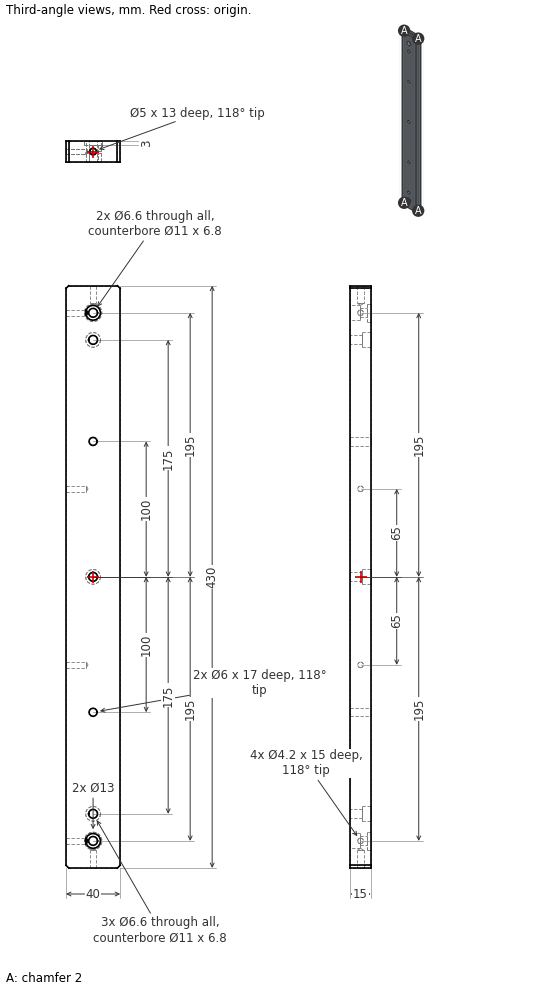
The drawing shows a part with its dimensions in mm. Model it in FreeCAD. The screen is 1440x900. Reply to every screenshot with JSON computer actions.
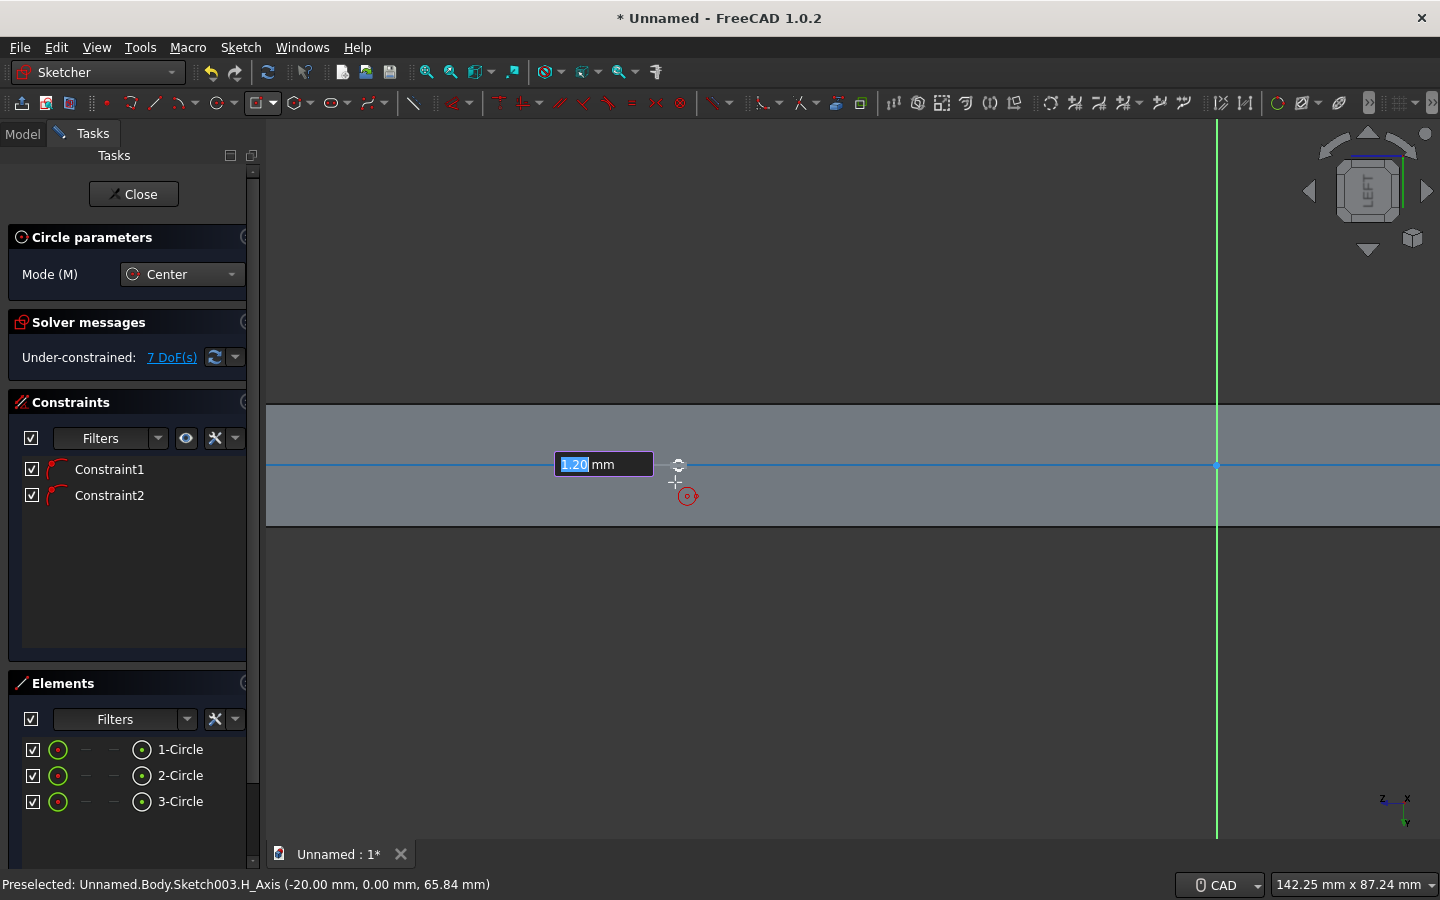
{"action": "left_click", "coordinate": [675, 482]}
{"action": "key", "text": "Escape"}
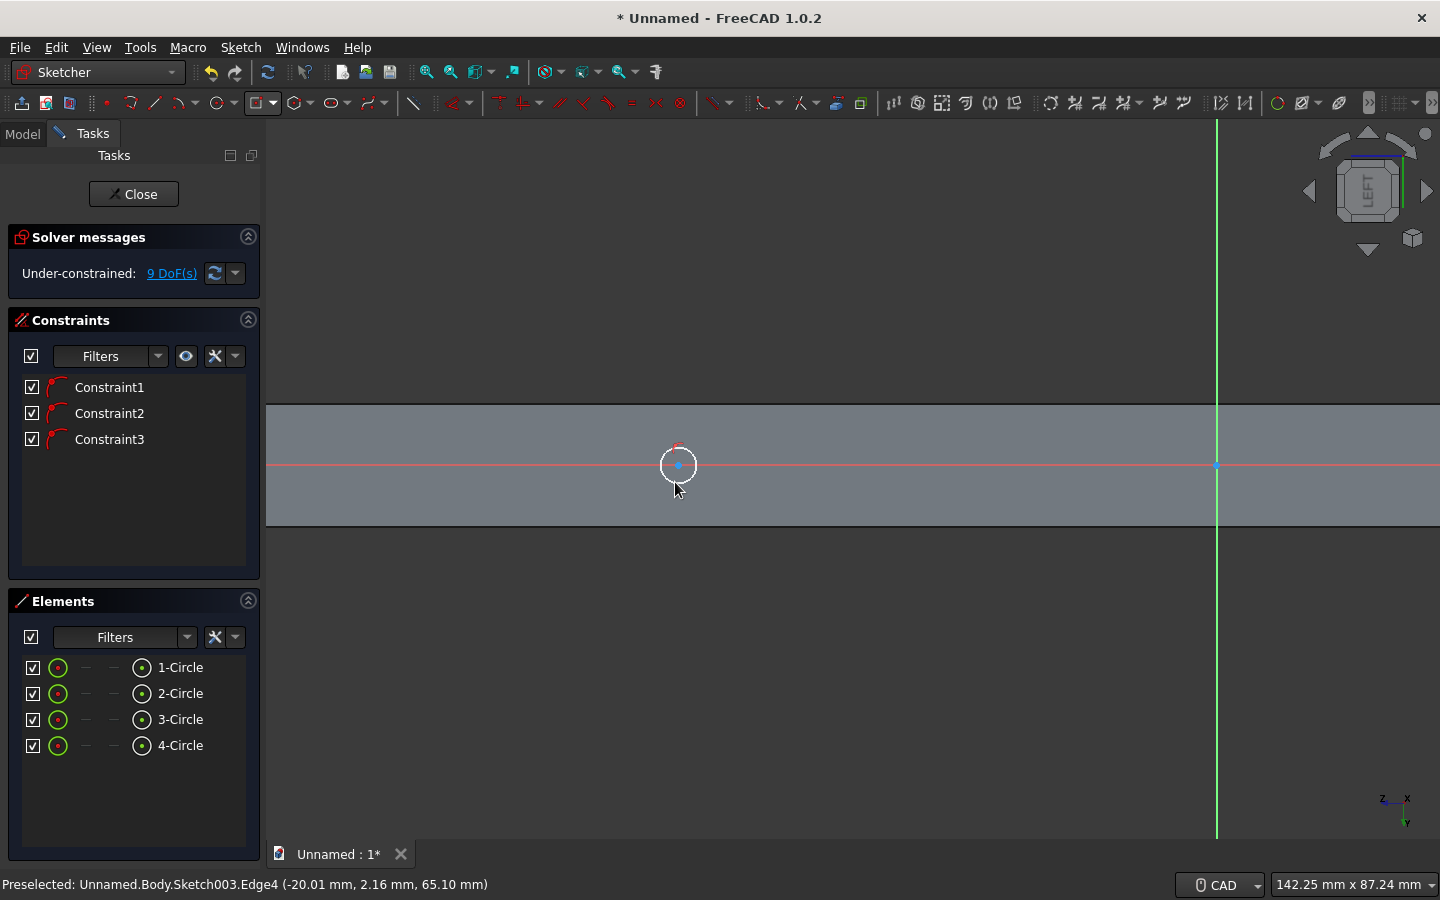
{"action": "scroll", "coordinate": [675, 482], "scroll_direction": "down", "scroll_amount": 8}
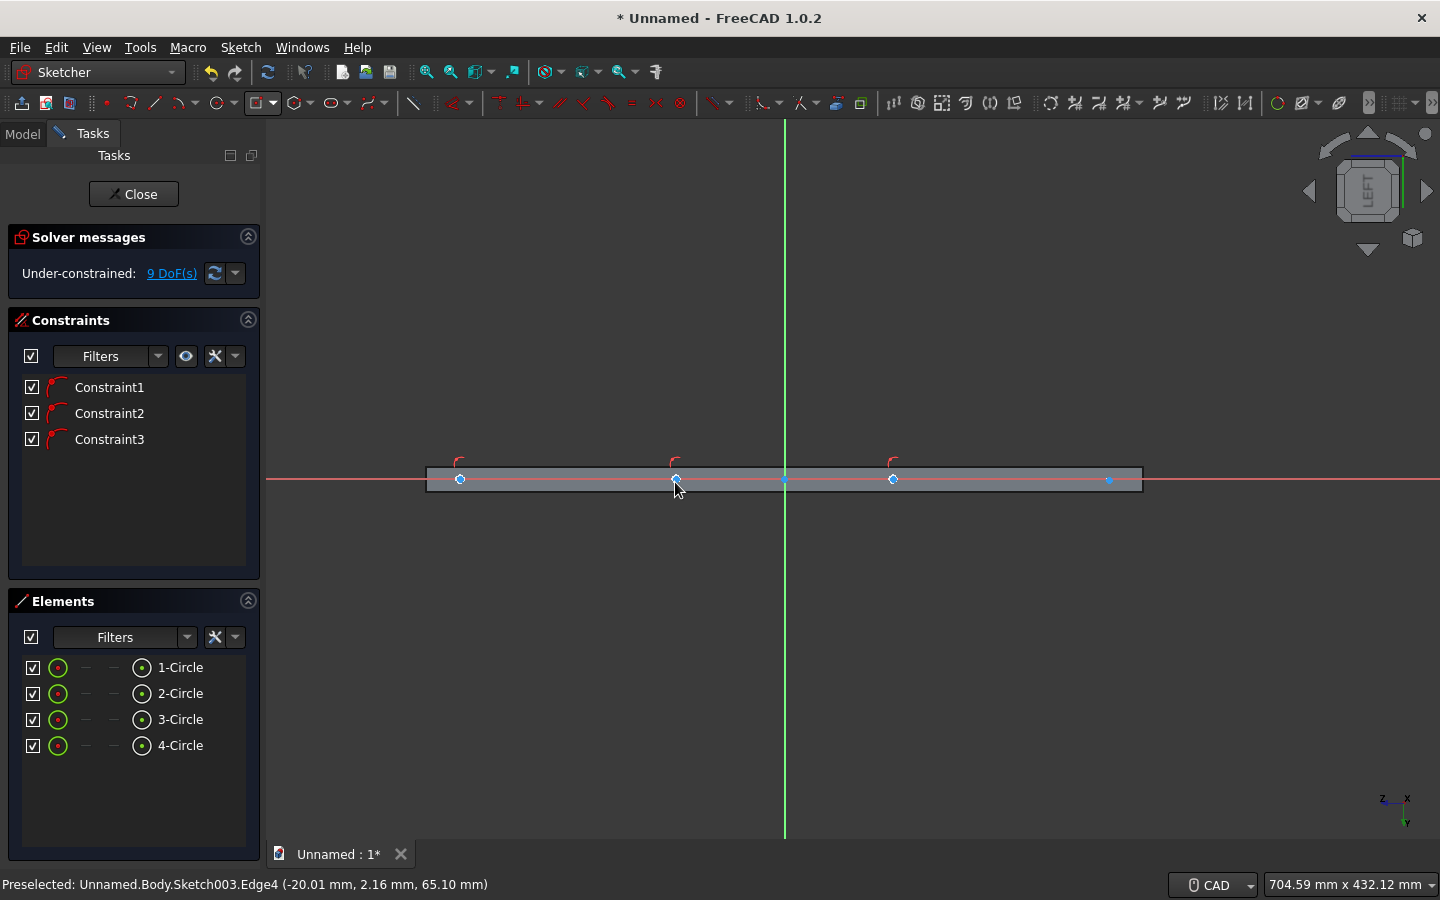
{"action": "scroll", "coordinate": [1111, 478], "scroll_direction": "up", "scroll_amount": 9}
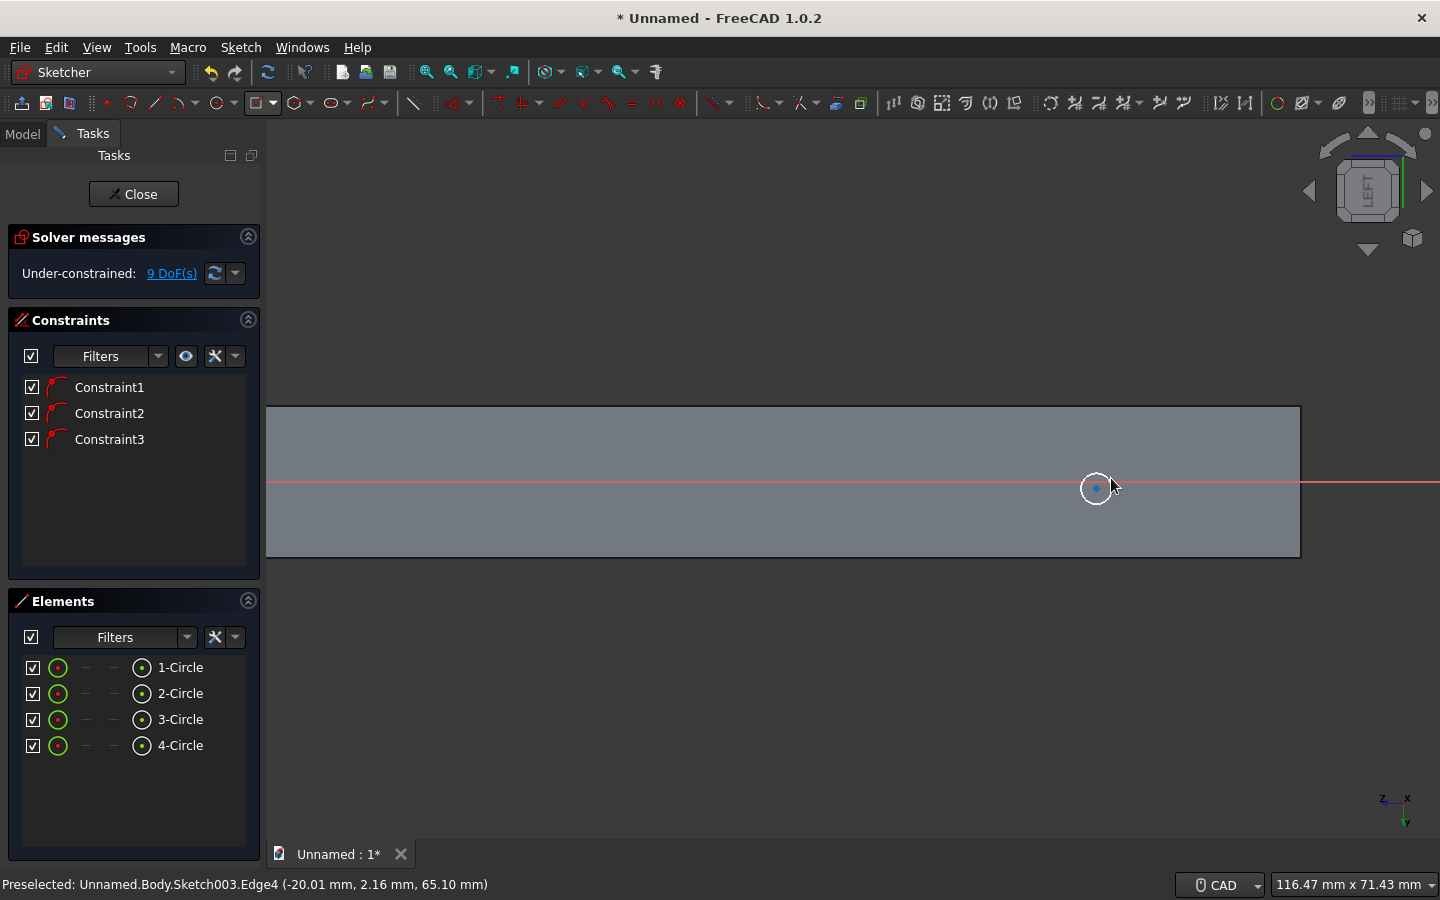
{"action": "left_click", "coordinate": [1107, 478]}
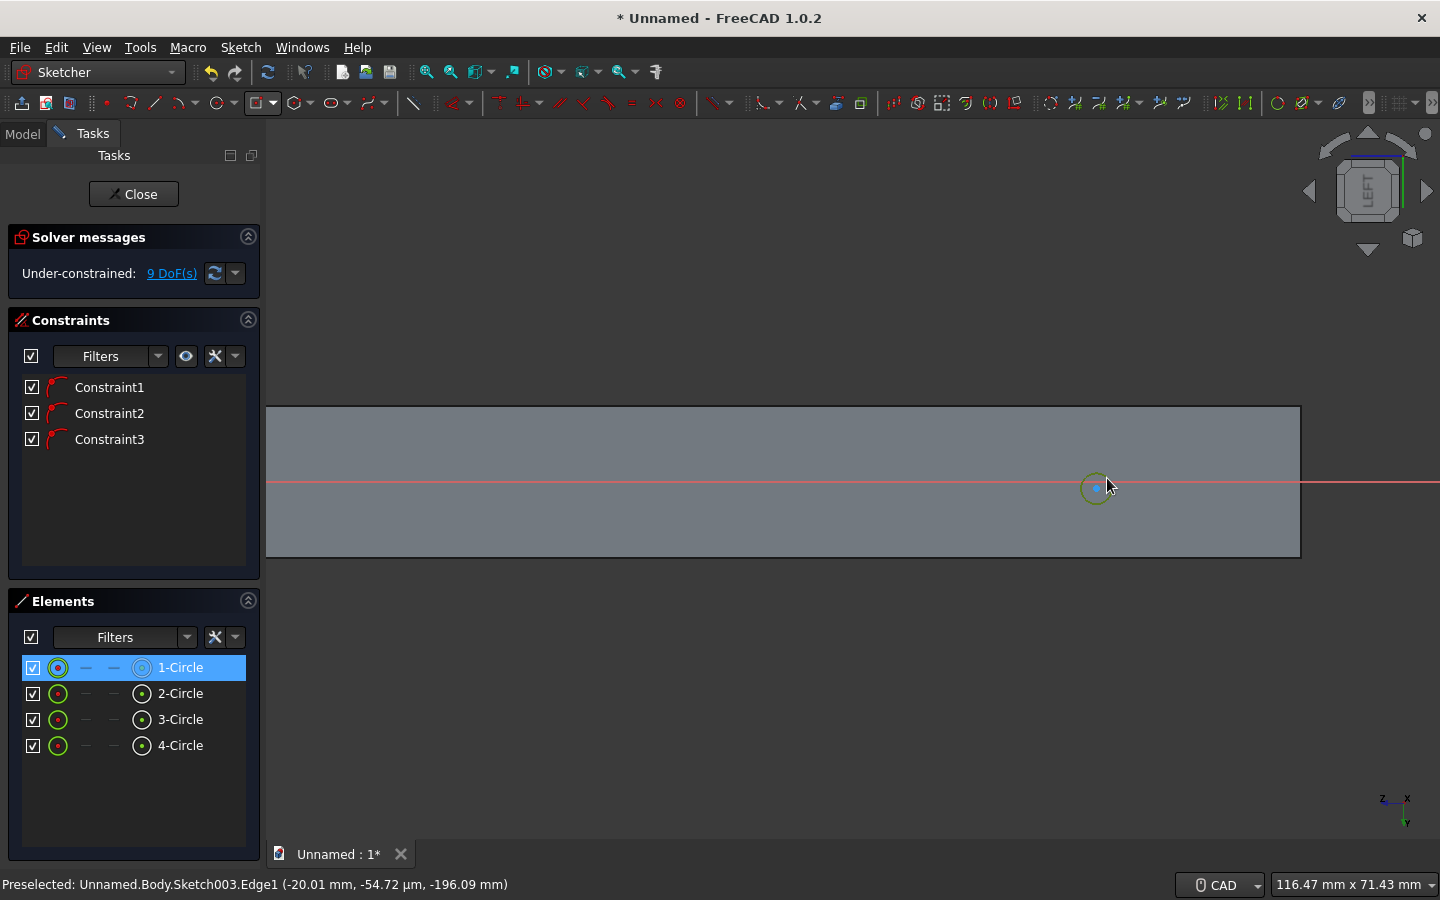
{"action": "scroll", "coordinate": [1111, 478], "scroll_direction": "down", "scroll_amount": 9}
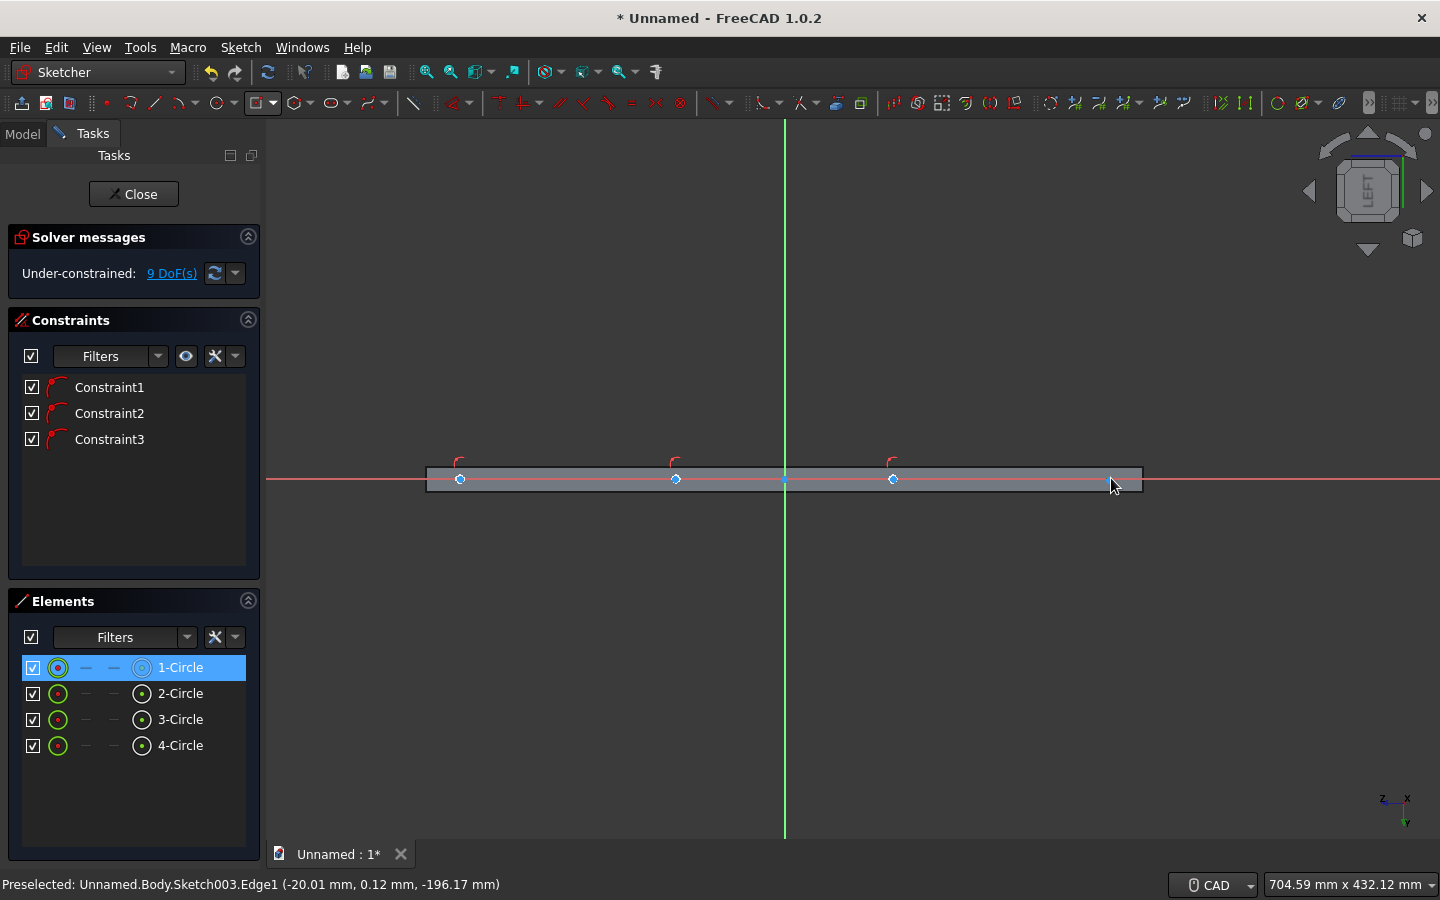
{"action": "scroll", "coordinate": [463, 476], "scroll_direction": "up", "scroll_amount": 9}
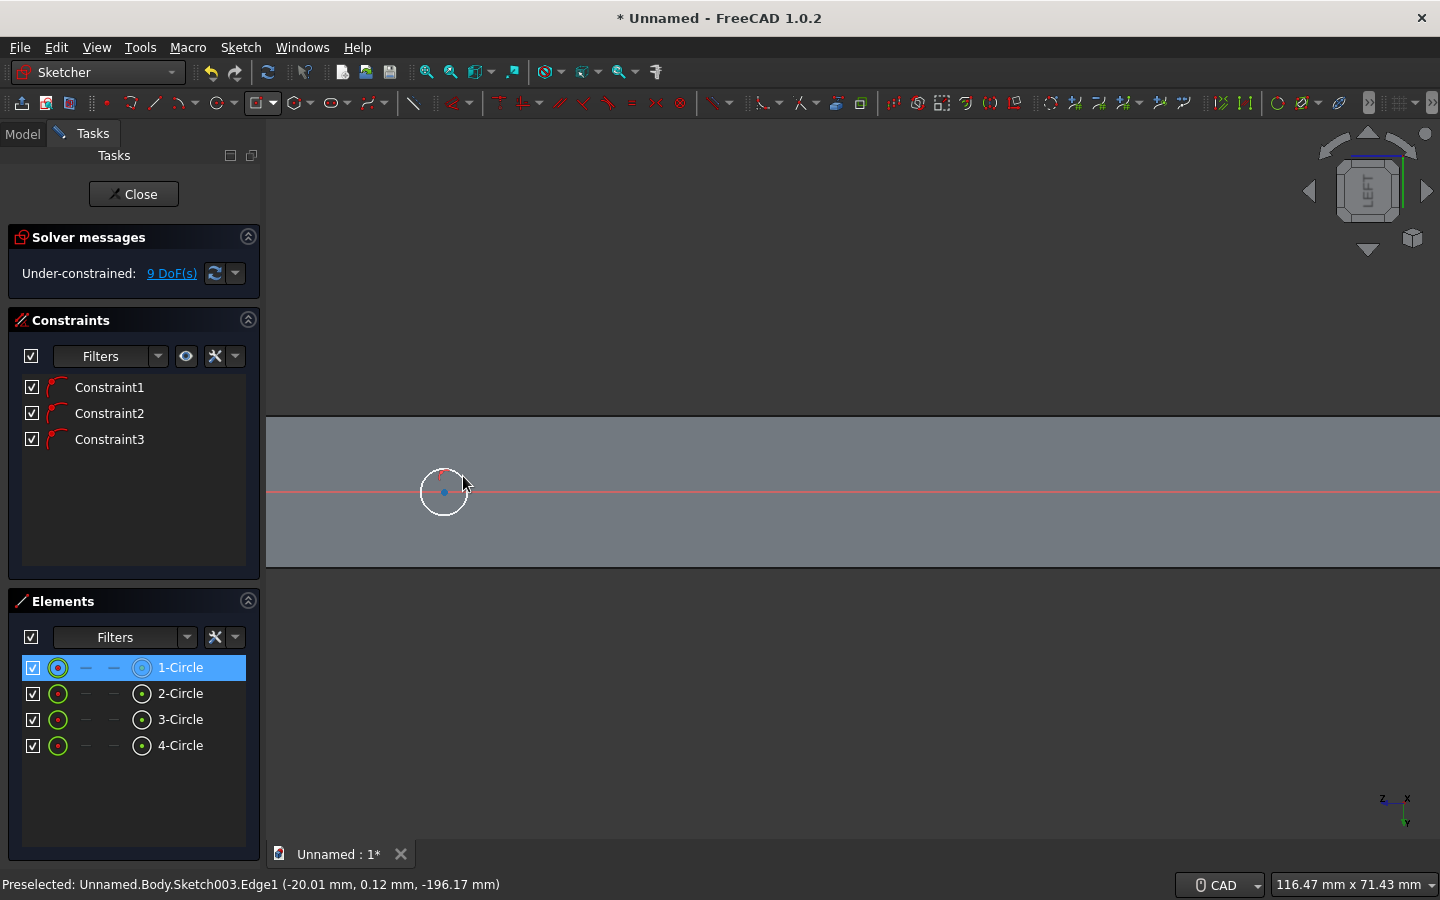
{"action": "left_click", "coordinate": [460, 476]}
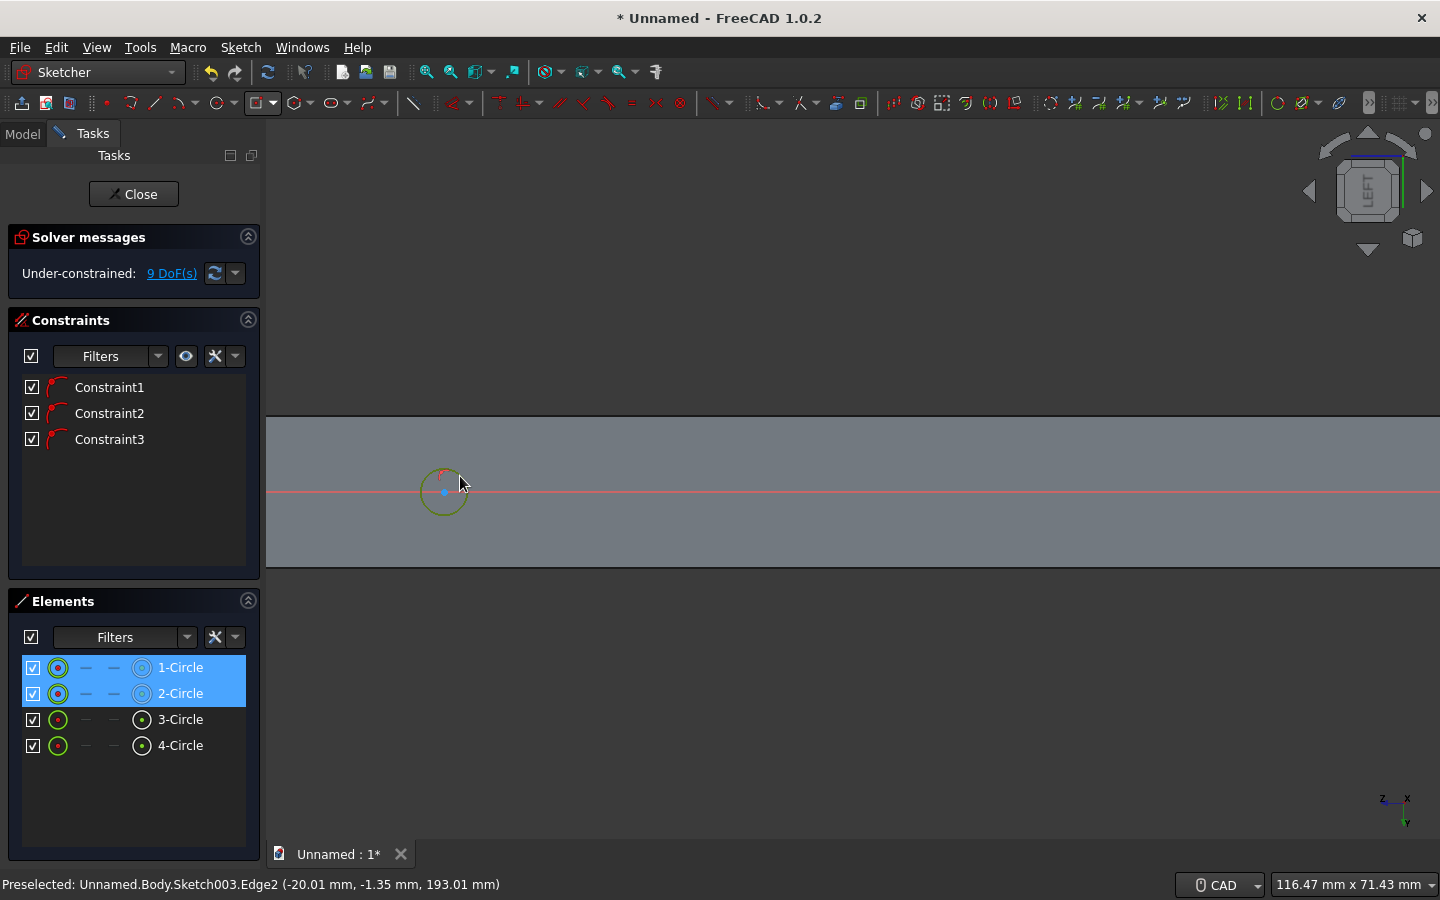
{"action": "scroll", "coordinate": [463, 476], "scroll_direction": "down", "scroll_amount": 9}